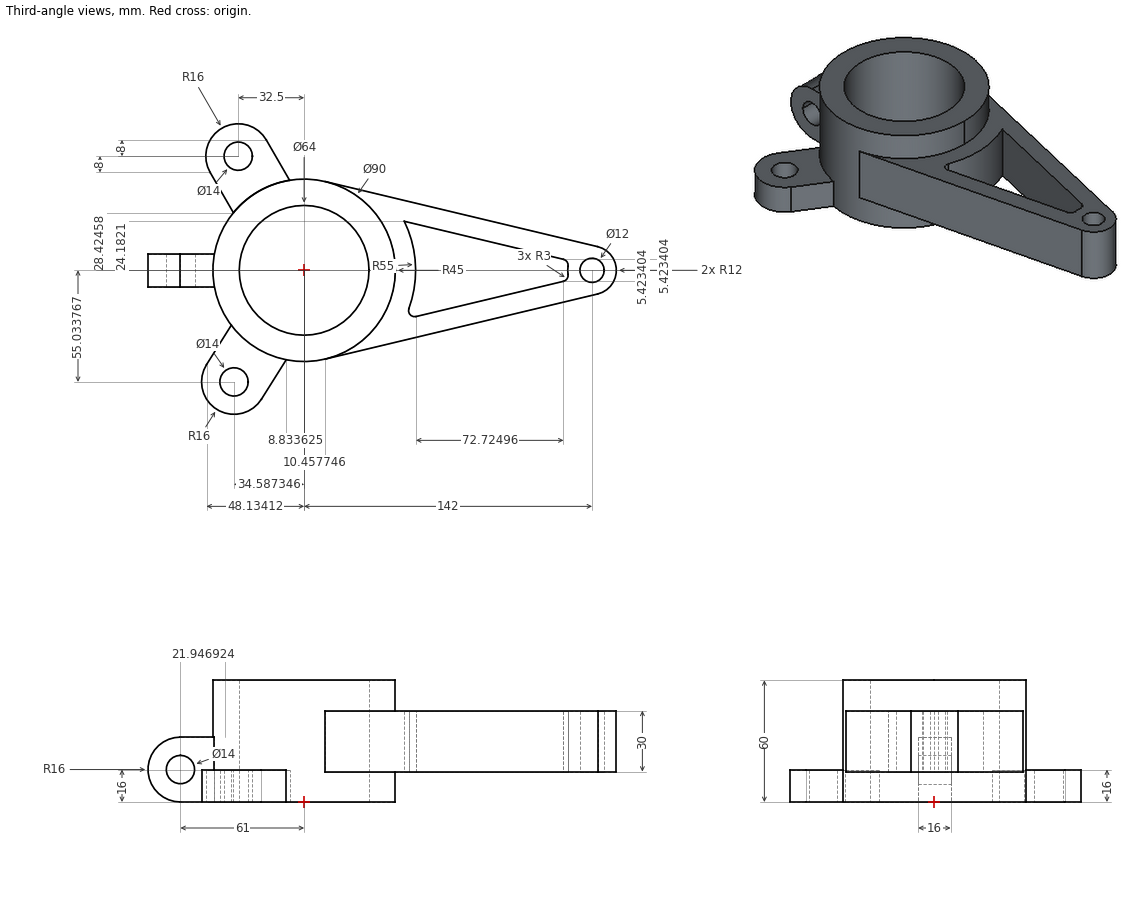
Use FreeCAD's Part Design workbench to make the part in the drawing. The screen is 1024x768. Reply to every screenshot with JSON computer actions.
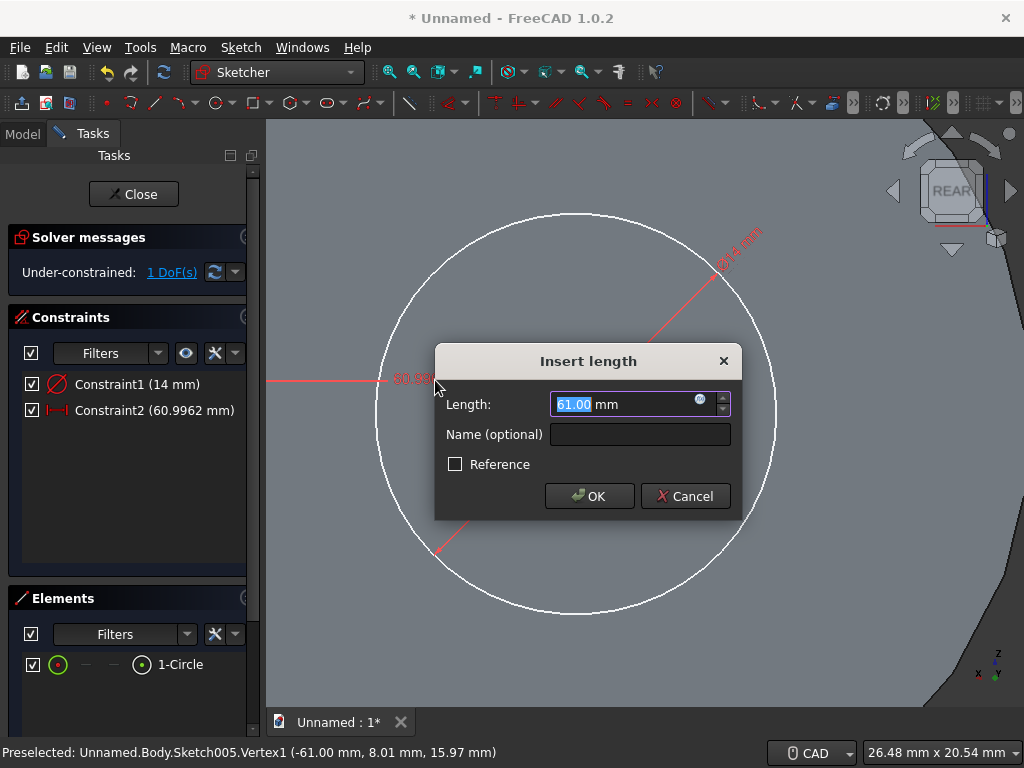
{"action": "type", "text": "61"}
{"action": "key", "text": "Return"}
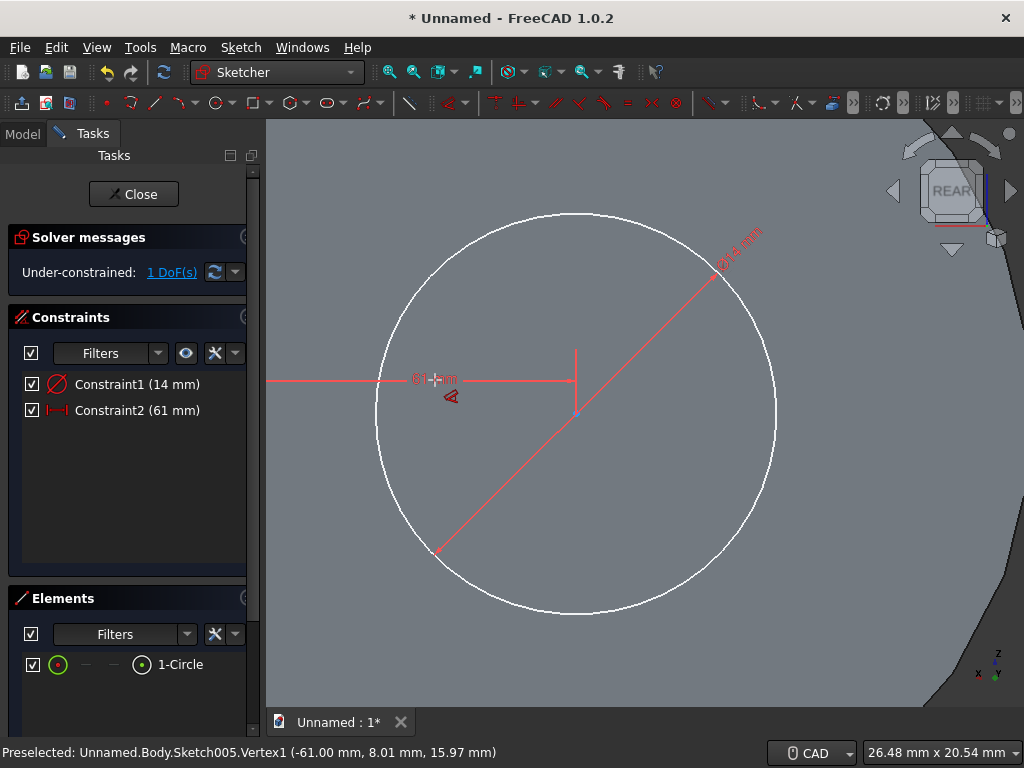
{"action": "left_click", "coordinate": [576, 414]}
{"action": "left_click", "coordinate": [610, 546]}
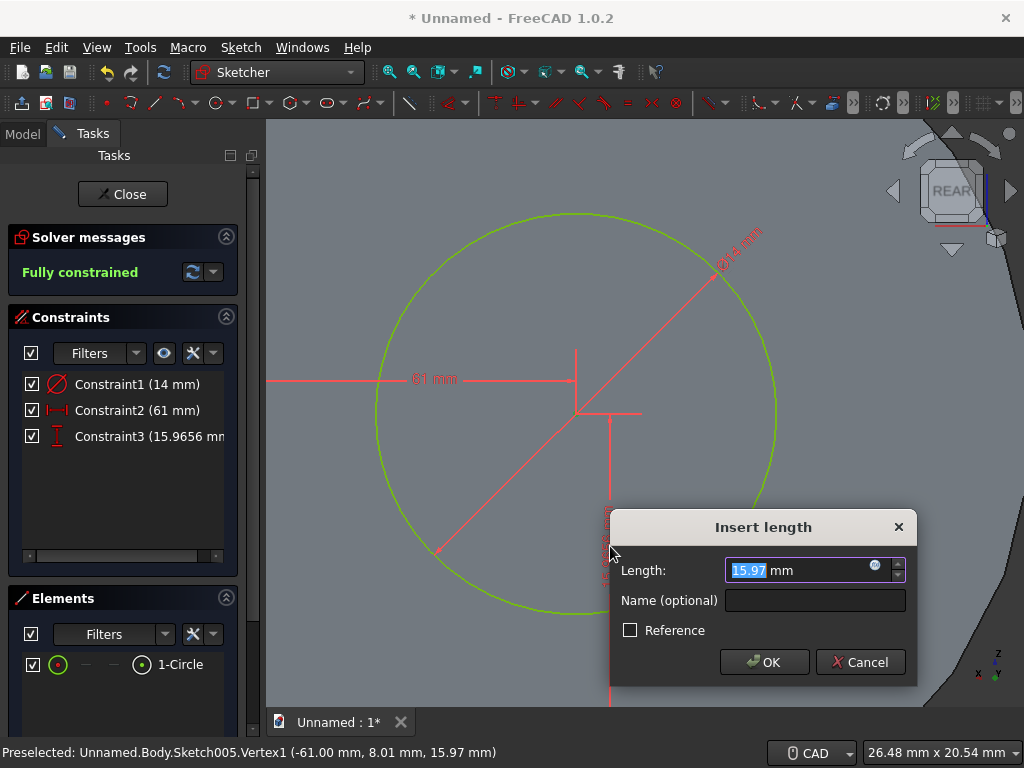
{"action": "type", "text": "16"}
{"action": "key", "text": "Return"}
{"action": "key", "text": "Escape"}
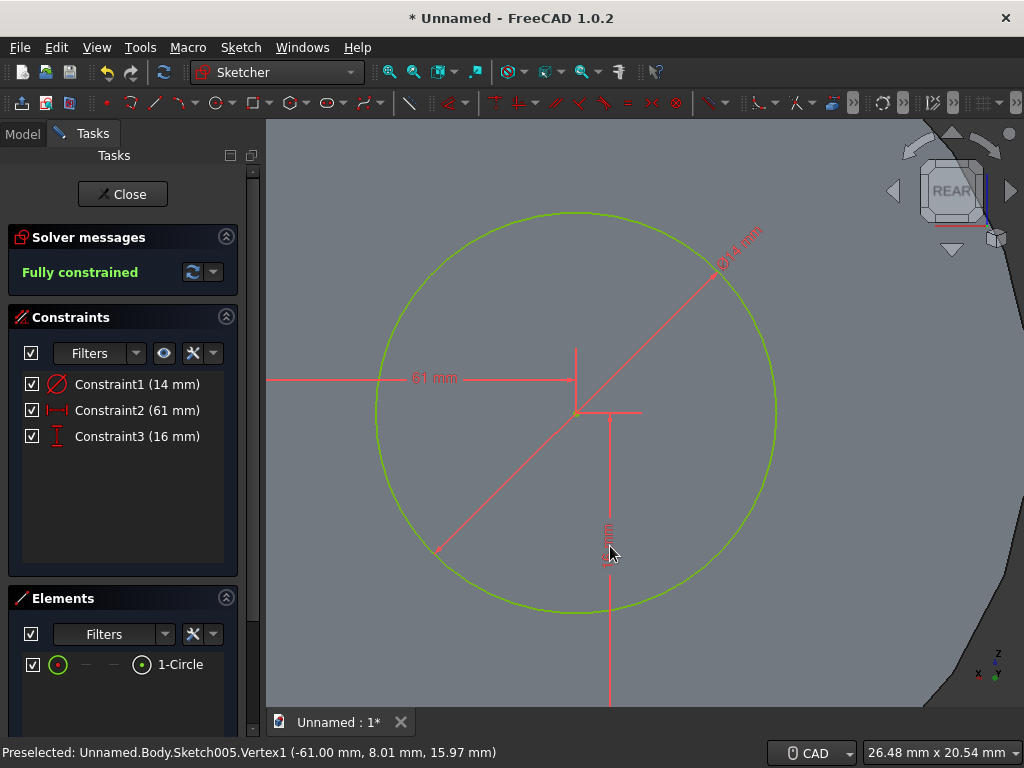
{"action": "left_click", "coordinate": [123, 194]}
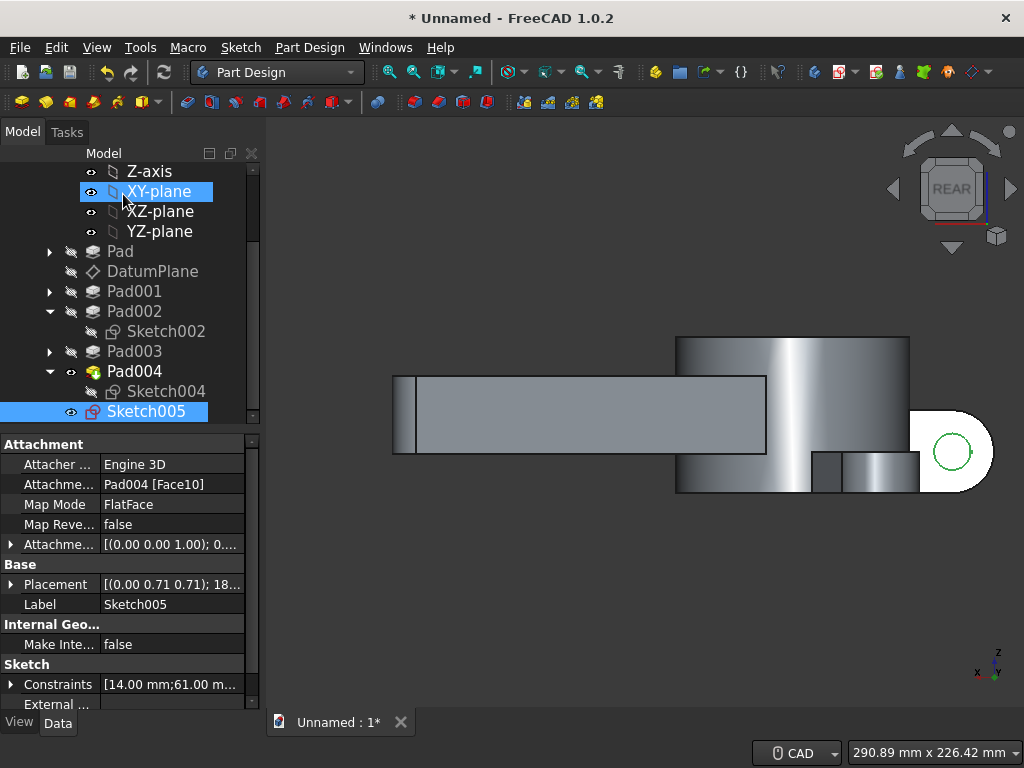
{"action": "left_click", "coordinate": [188, 102]}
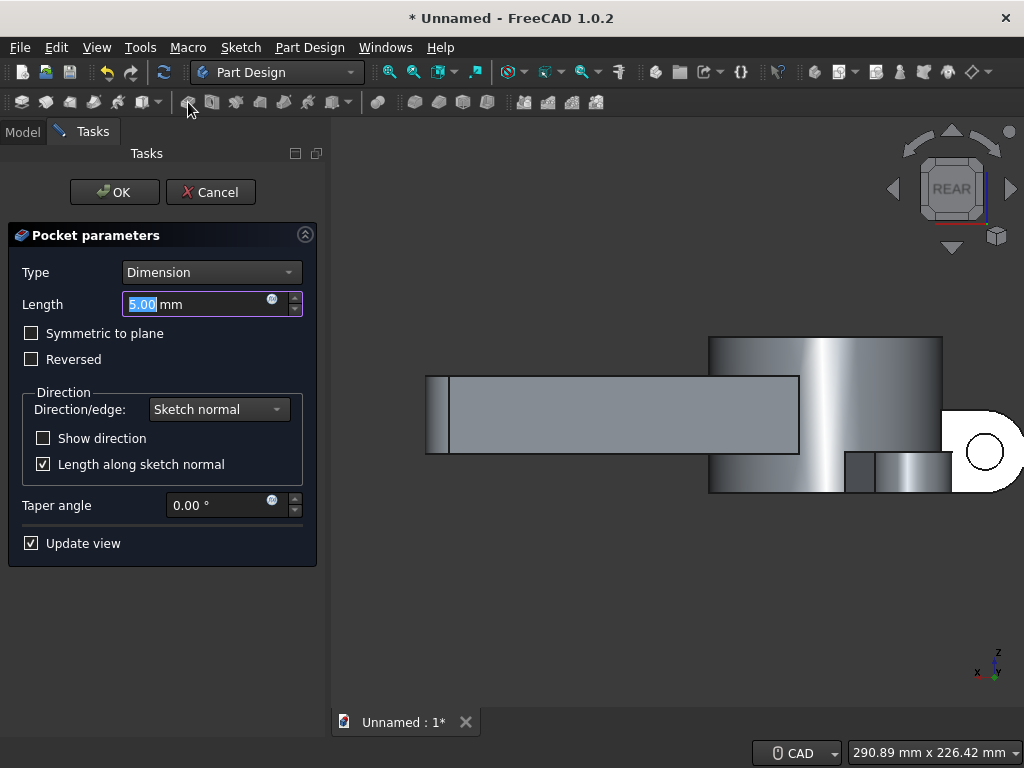
{"action": "type", "text": "16"}
{"action": "key", "text": "Tab"}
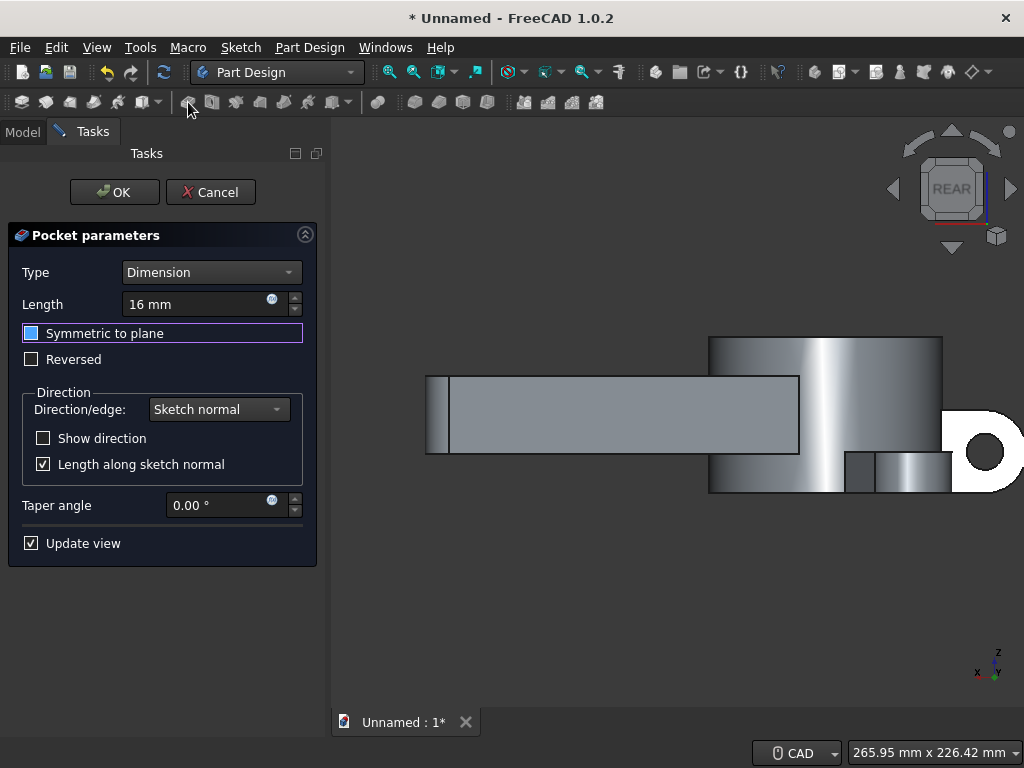
{"action": "left_click", "coordinate": [115, 192]}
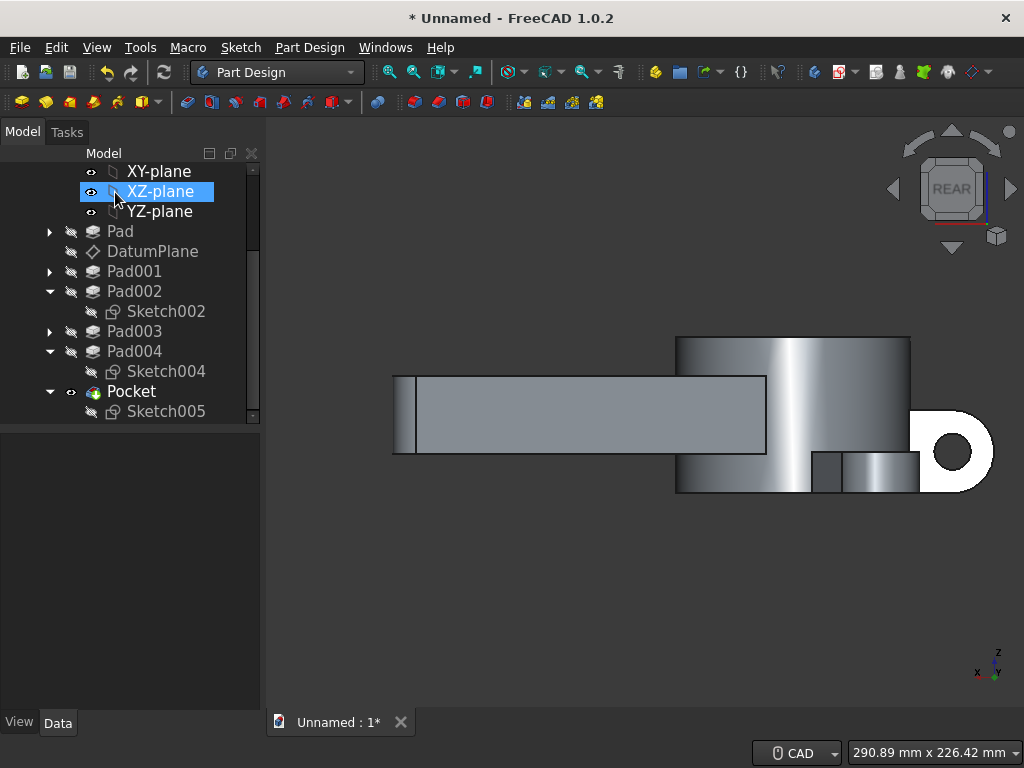
{"action": "key", "text": "0"}